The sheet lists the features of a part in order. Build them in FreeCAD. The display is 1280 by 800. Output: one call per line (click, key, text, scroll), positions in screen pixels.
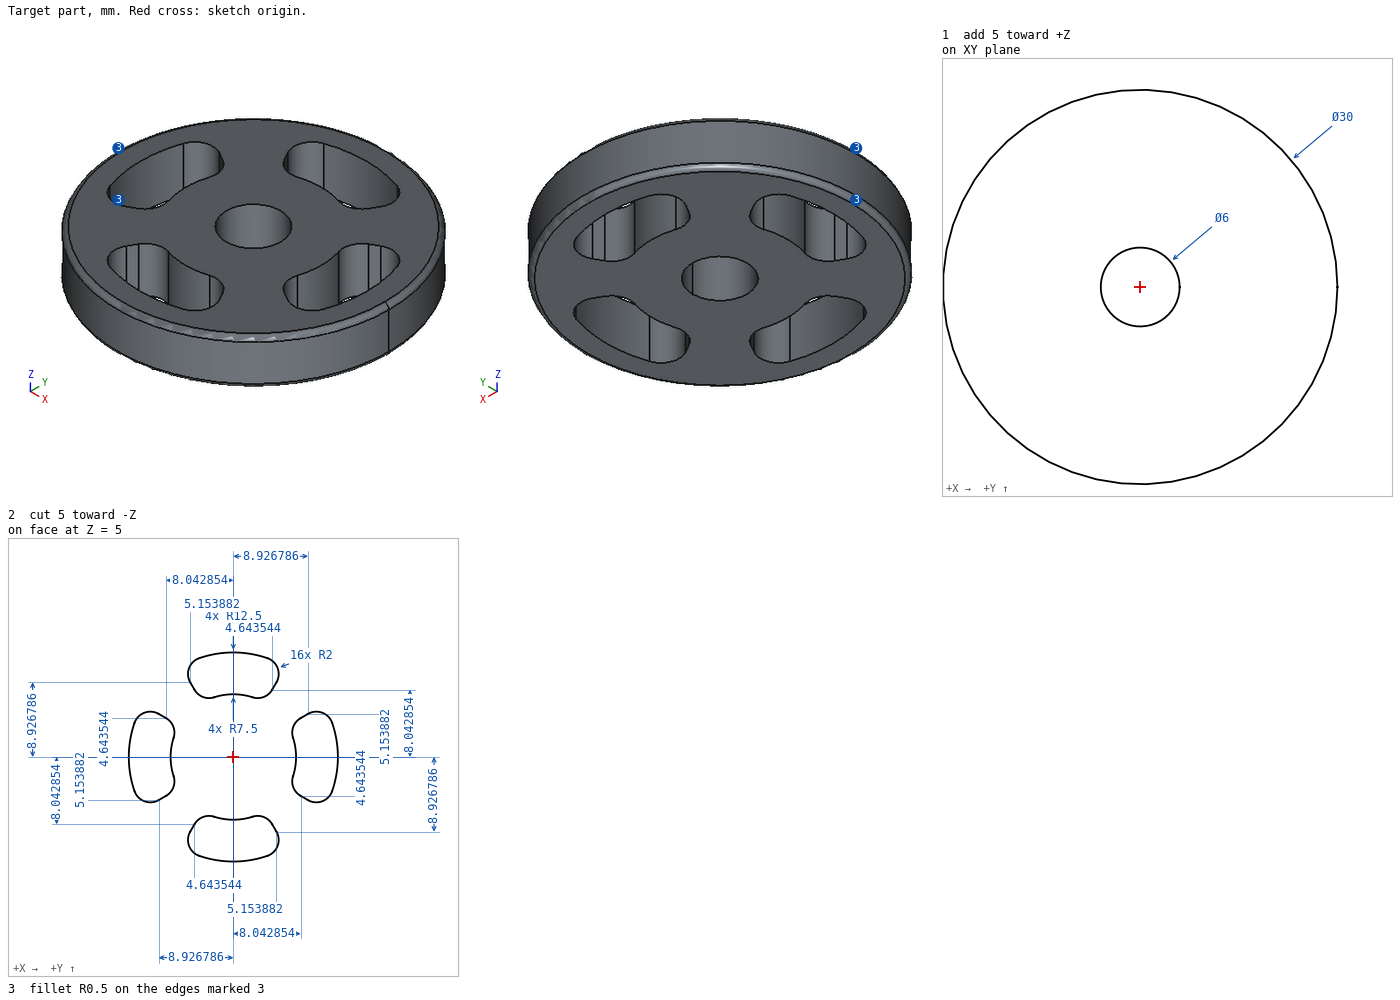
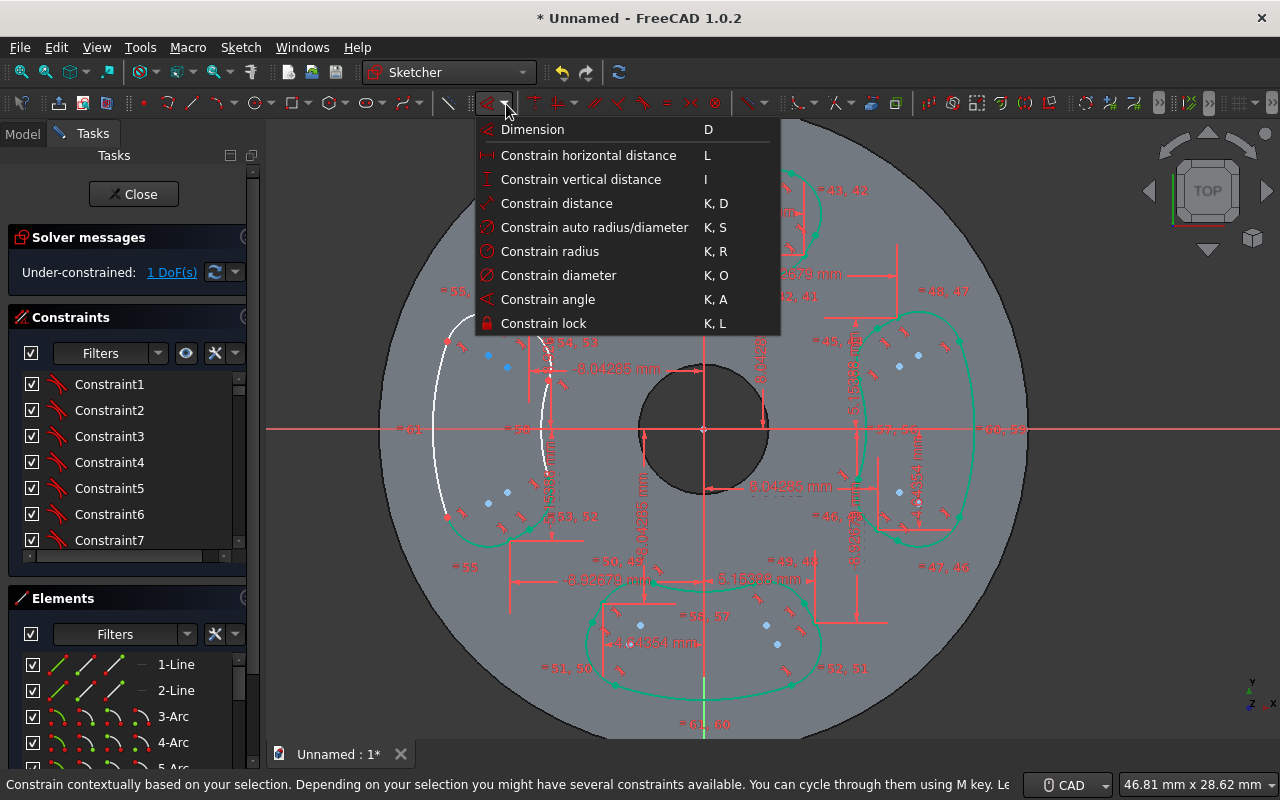
click(628, 179)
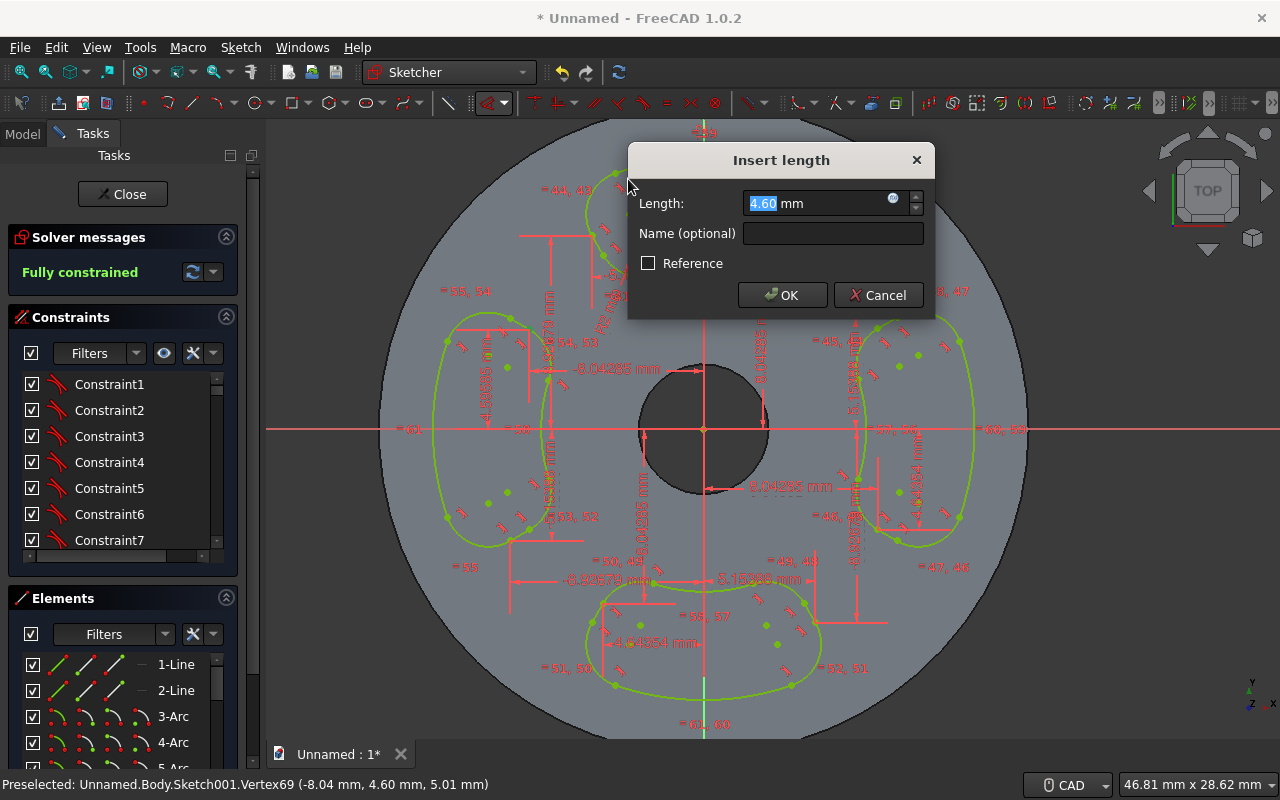
text(4.643544)
key(Return)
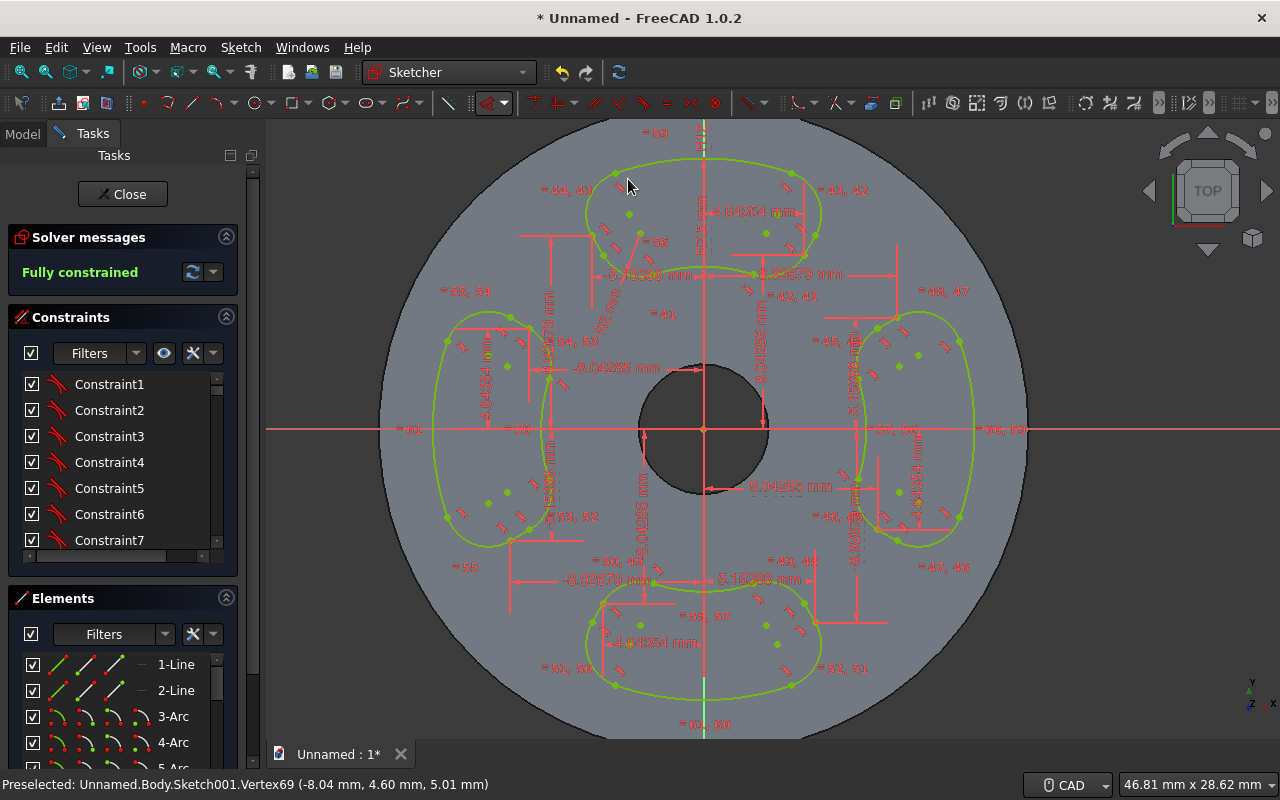
click(123, 194)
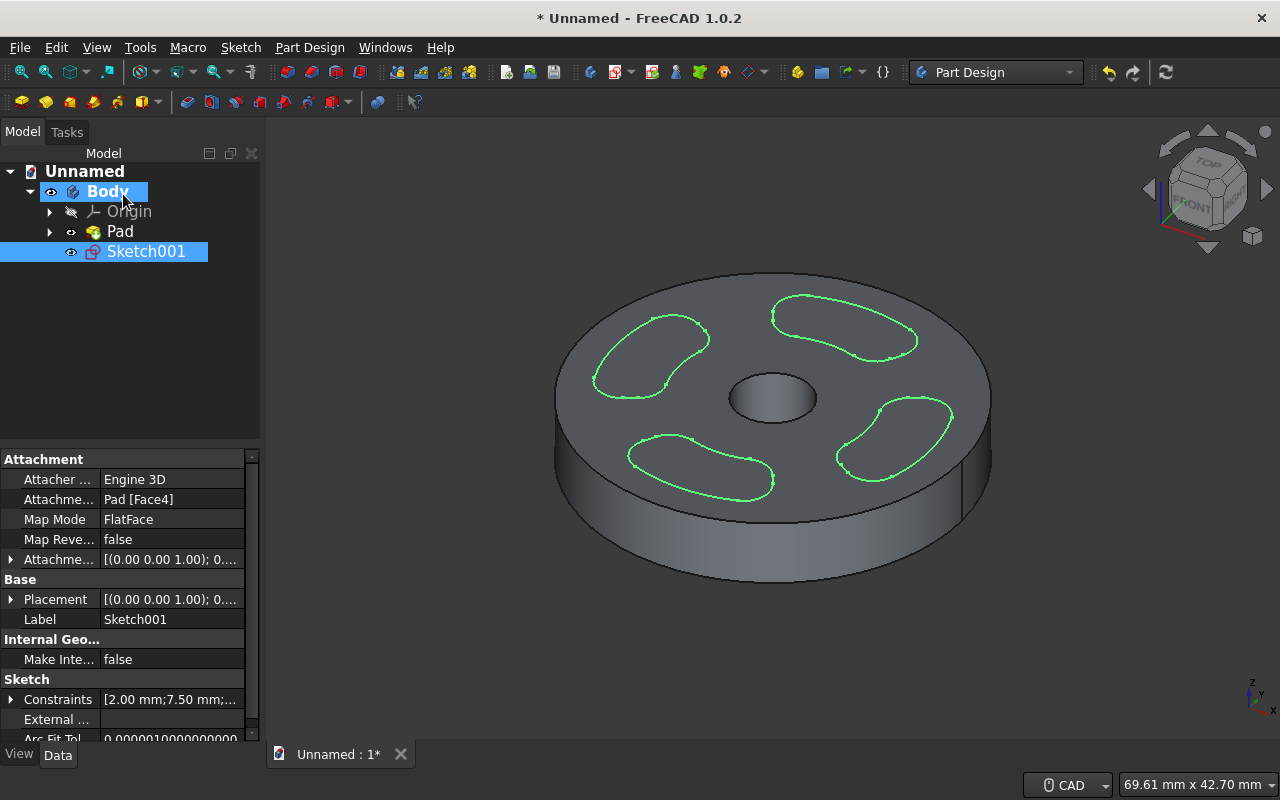
click(188, 102)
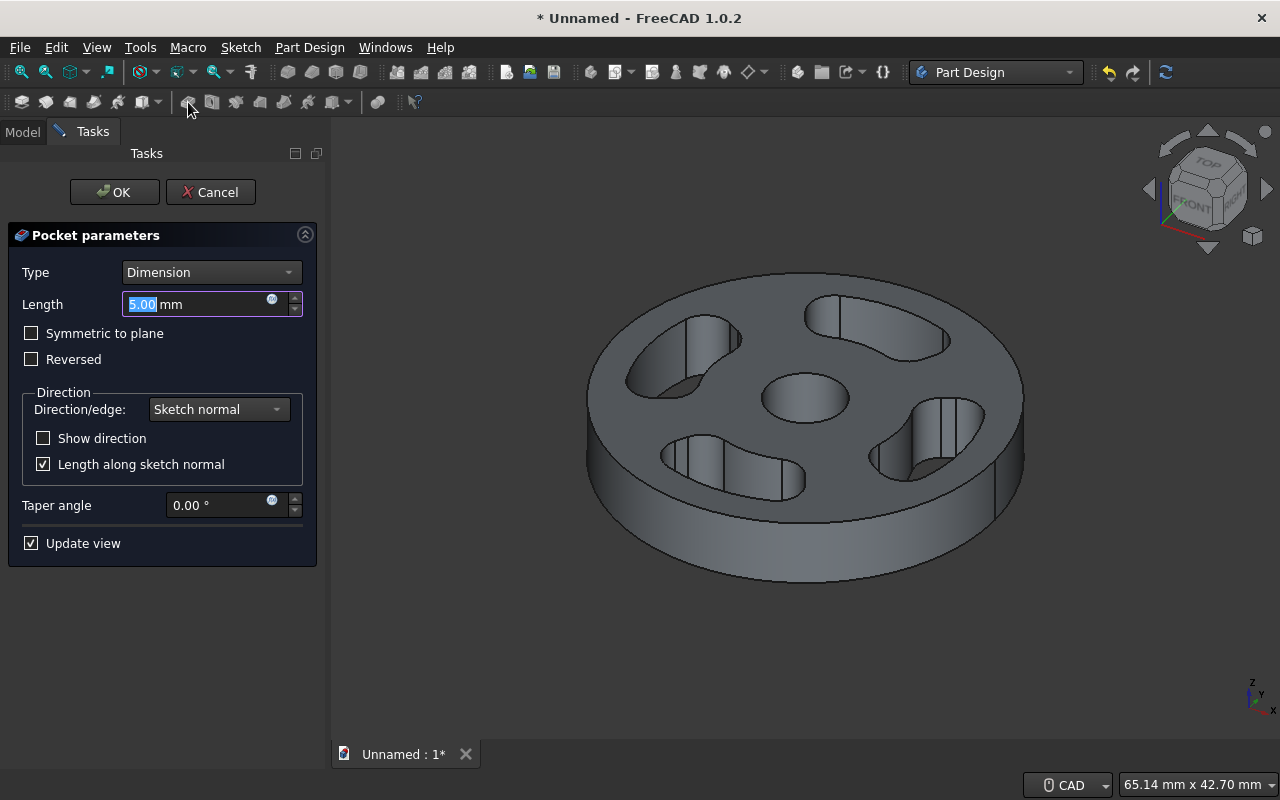
text(5)
key(Tab)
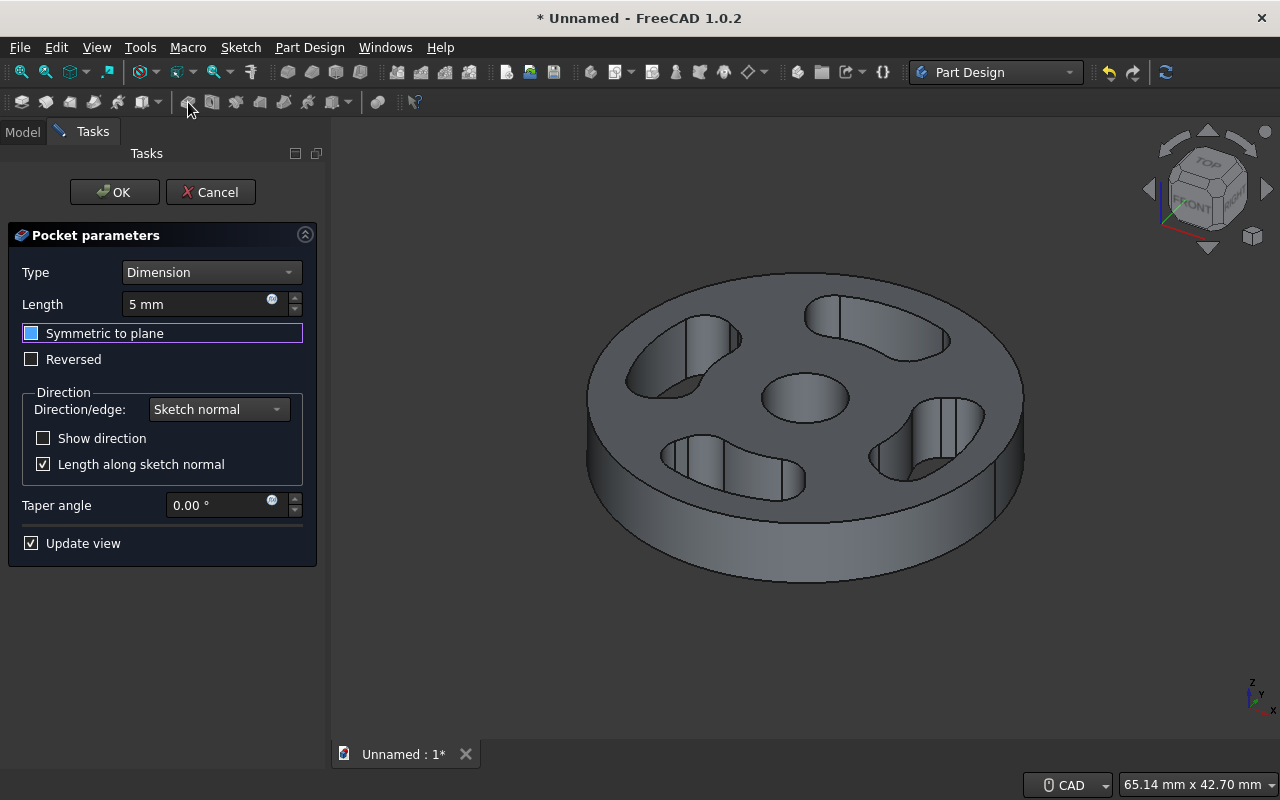
click(115, 192)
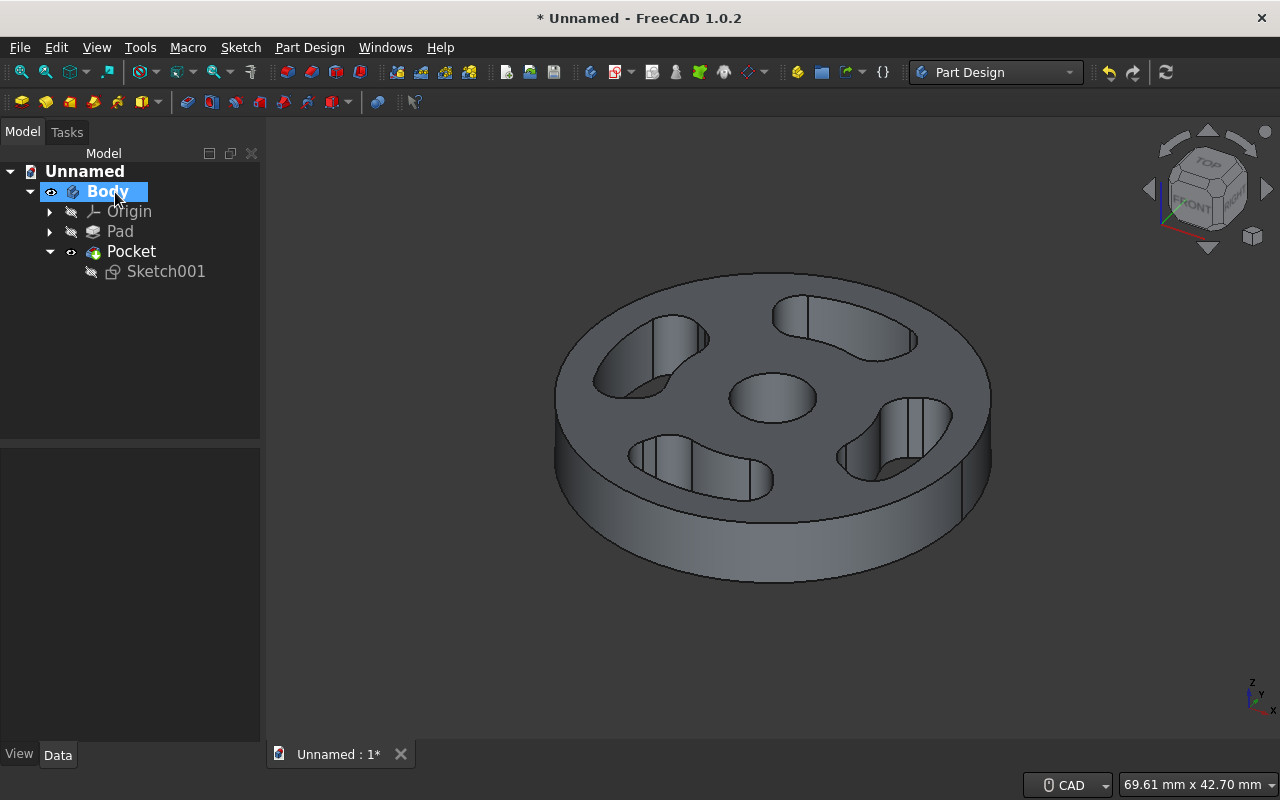
click(556, 410)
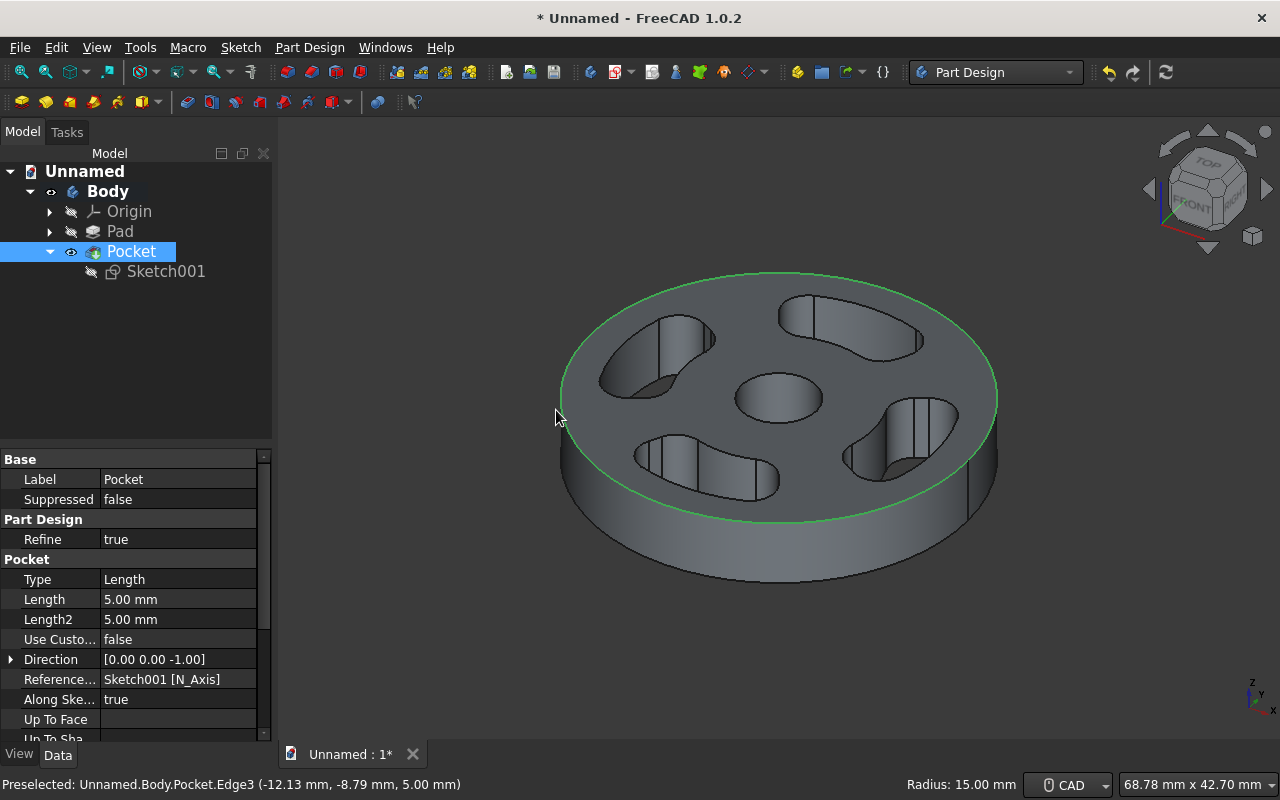
key(0)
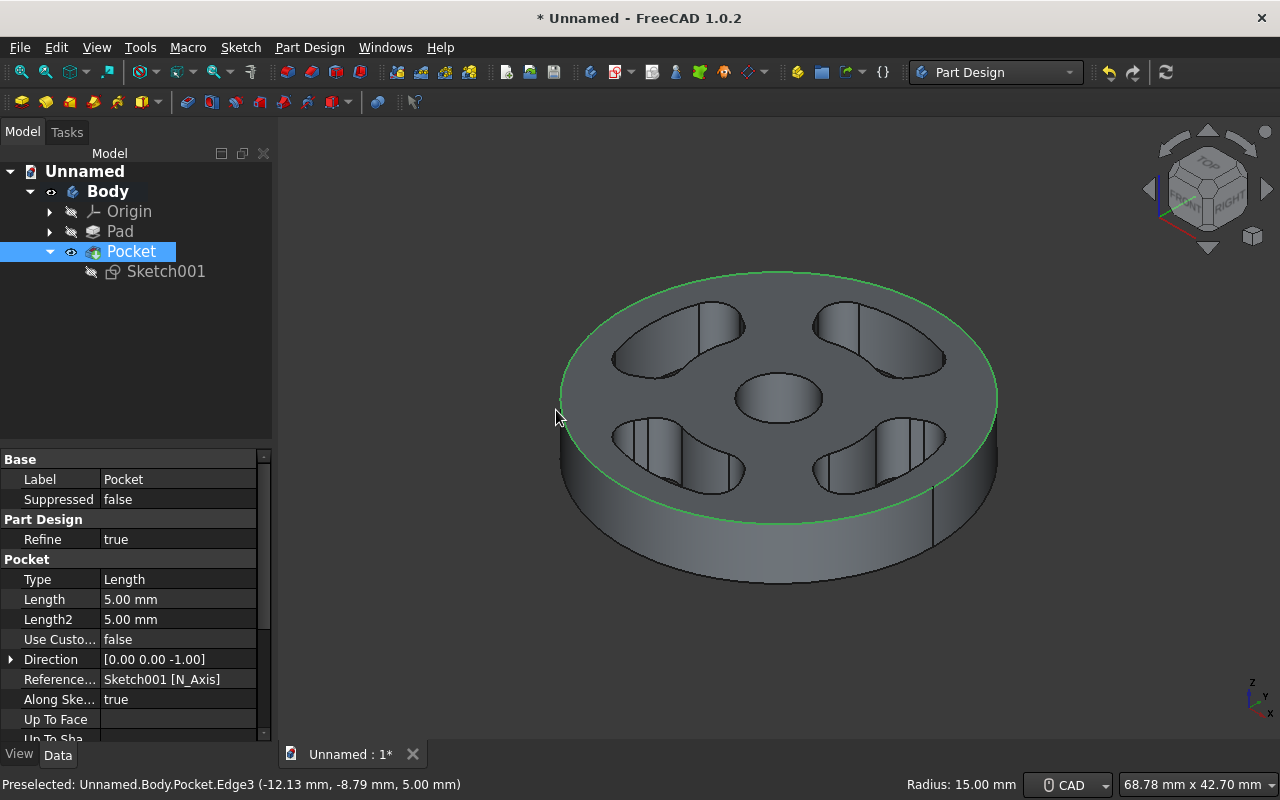
key(2)